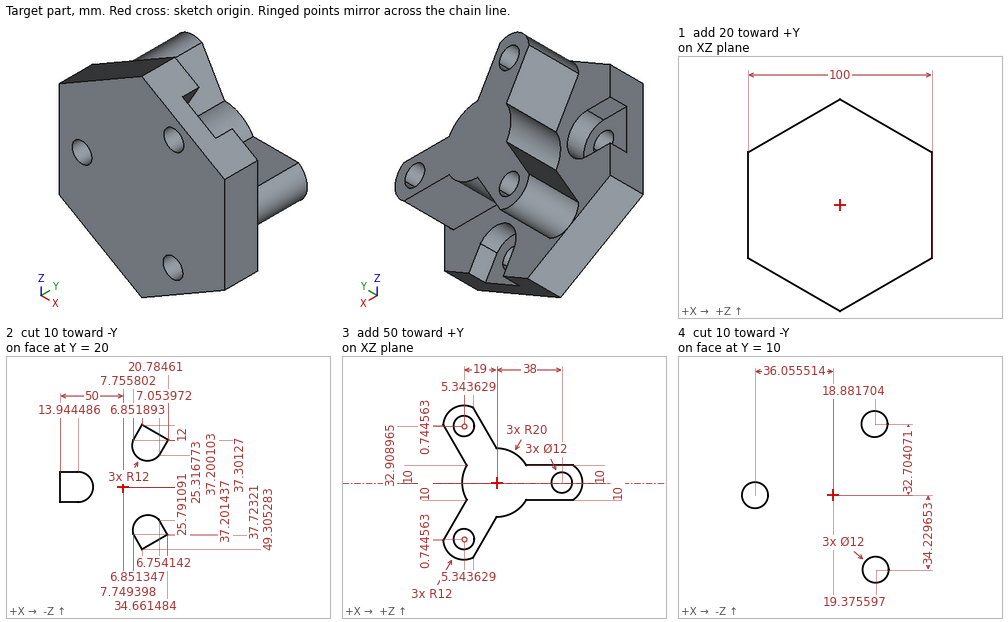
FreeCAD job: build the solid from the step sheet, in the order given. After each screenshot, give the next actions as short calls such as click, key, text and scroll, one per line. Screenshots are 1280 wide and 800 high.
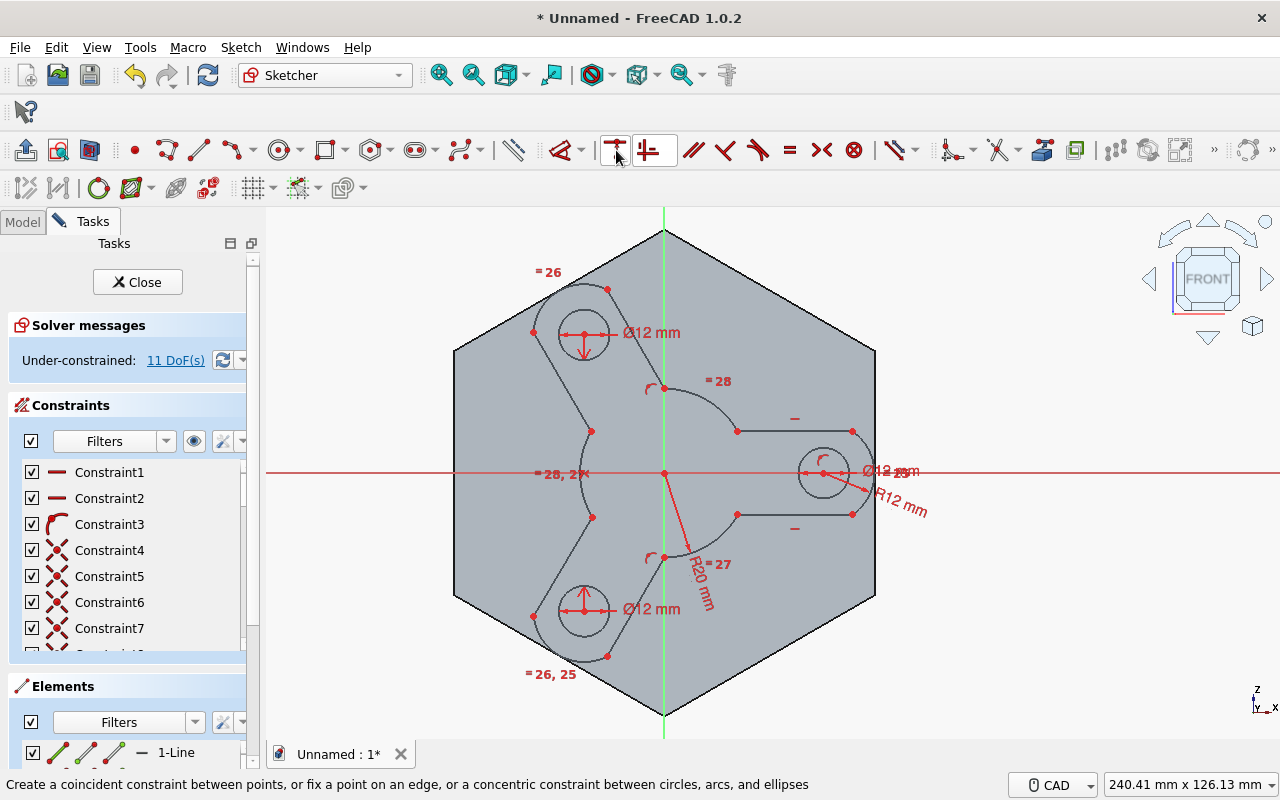
key(d)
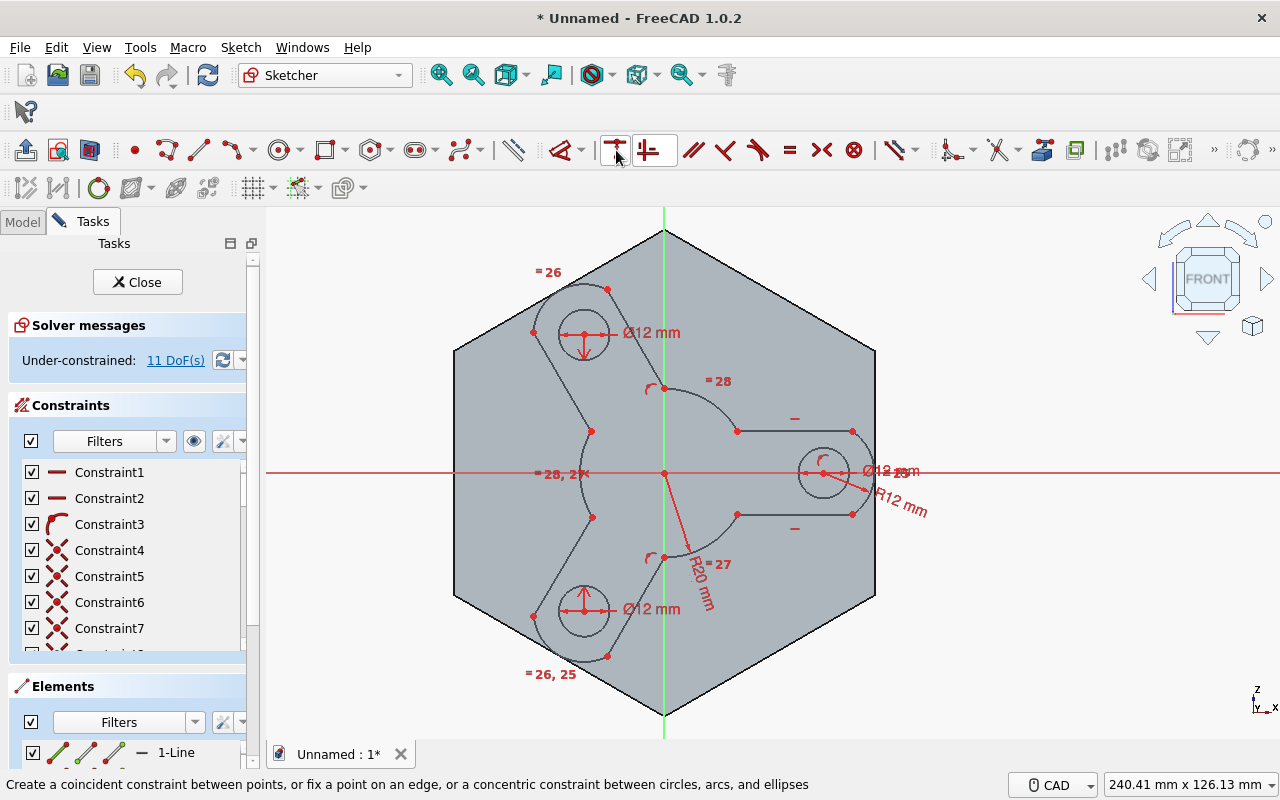
click(584, 335)
click(643, 301)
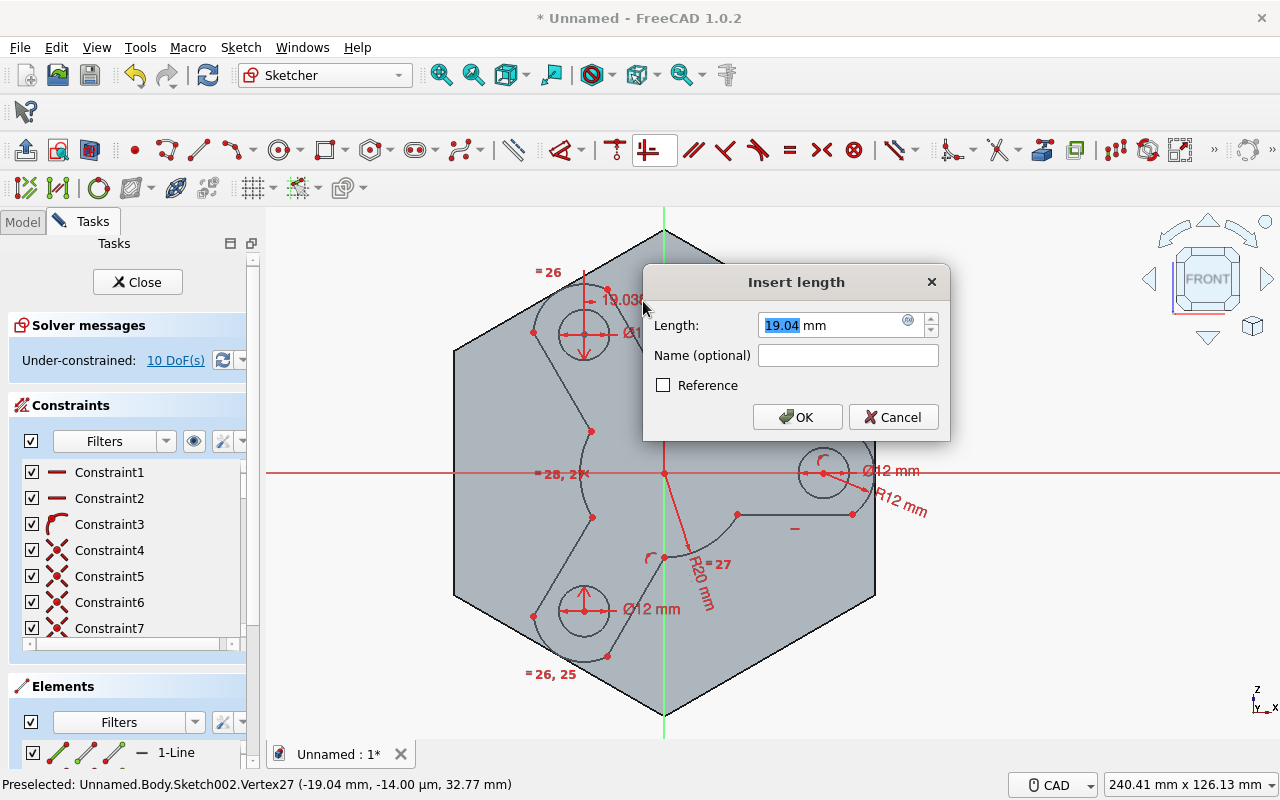
text(19)
key(Return)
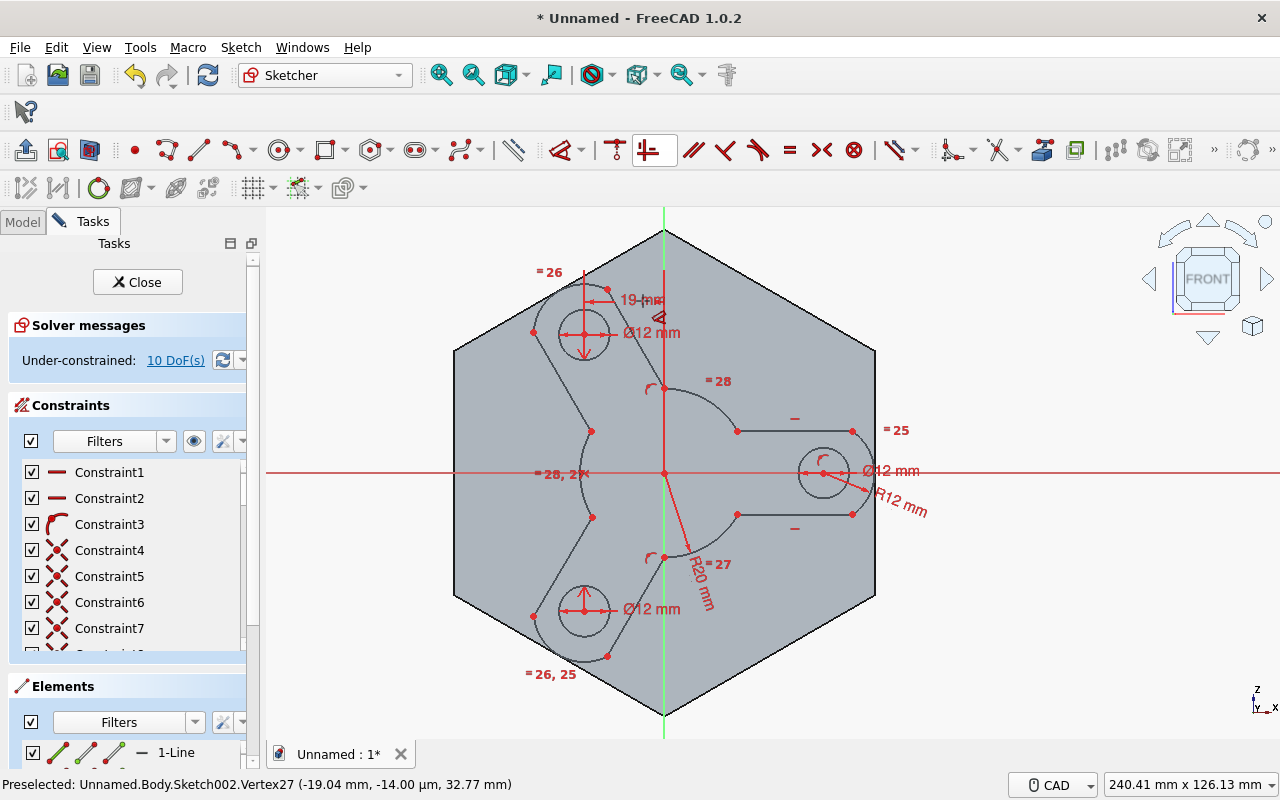
click(824, 473)
click(707, 507)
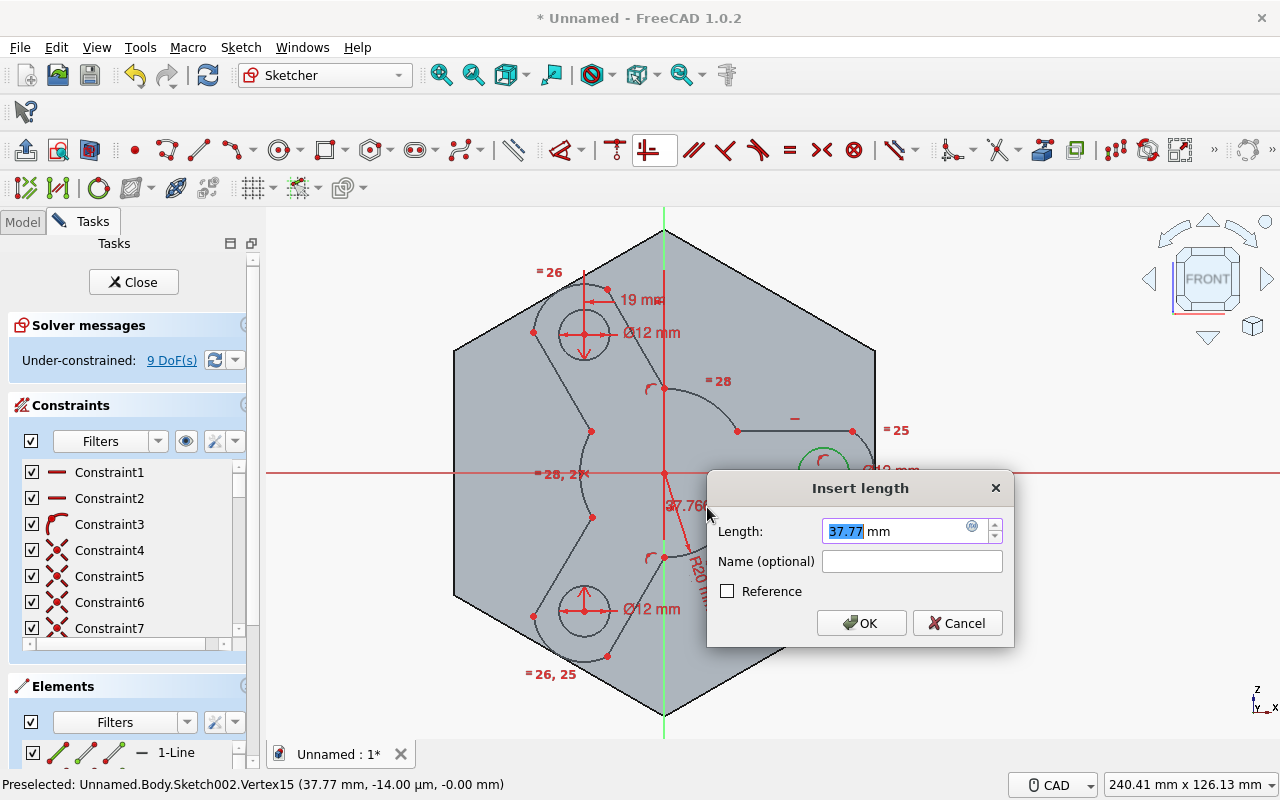
text(38)
key(Return)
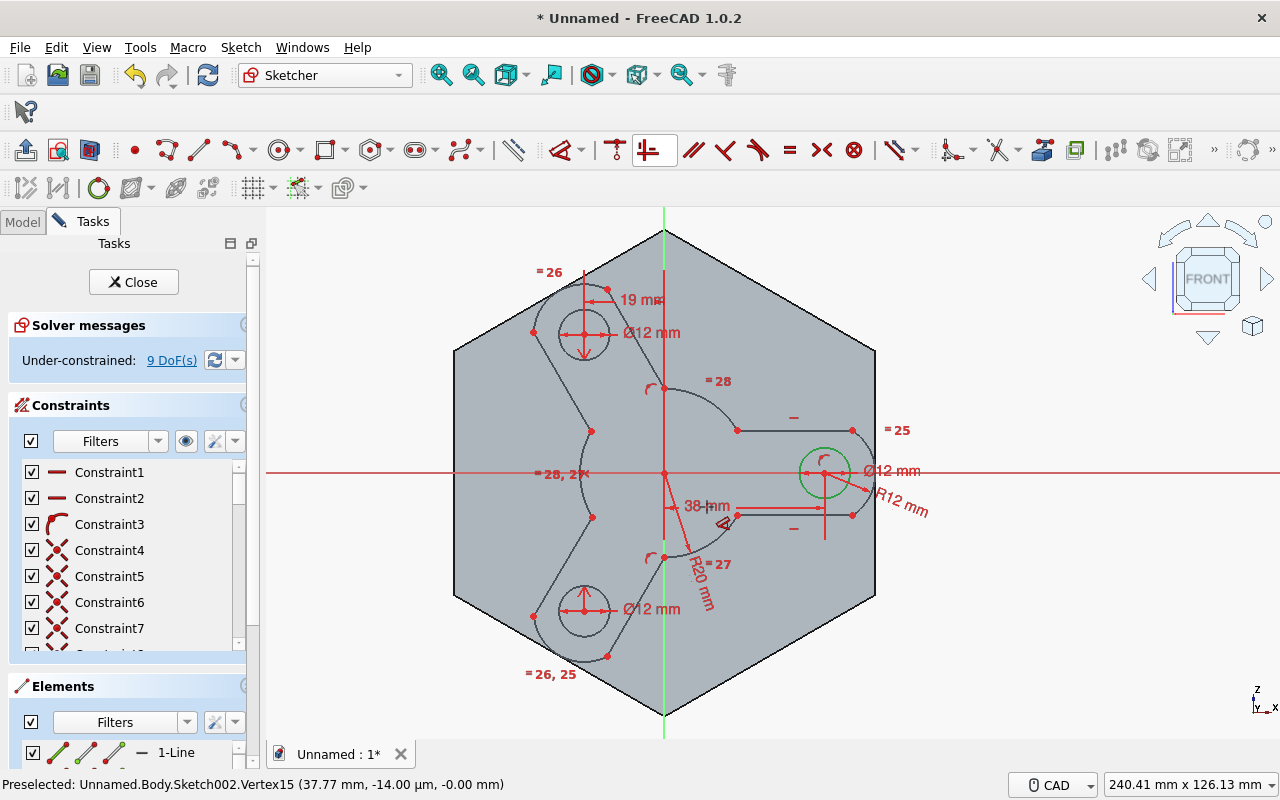
click(737, 431)
click(630, 452)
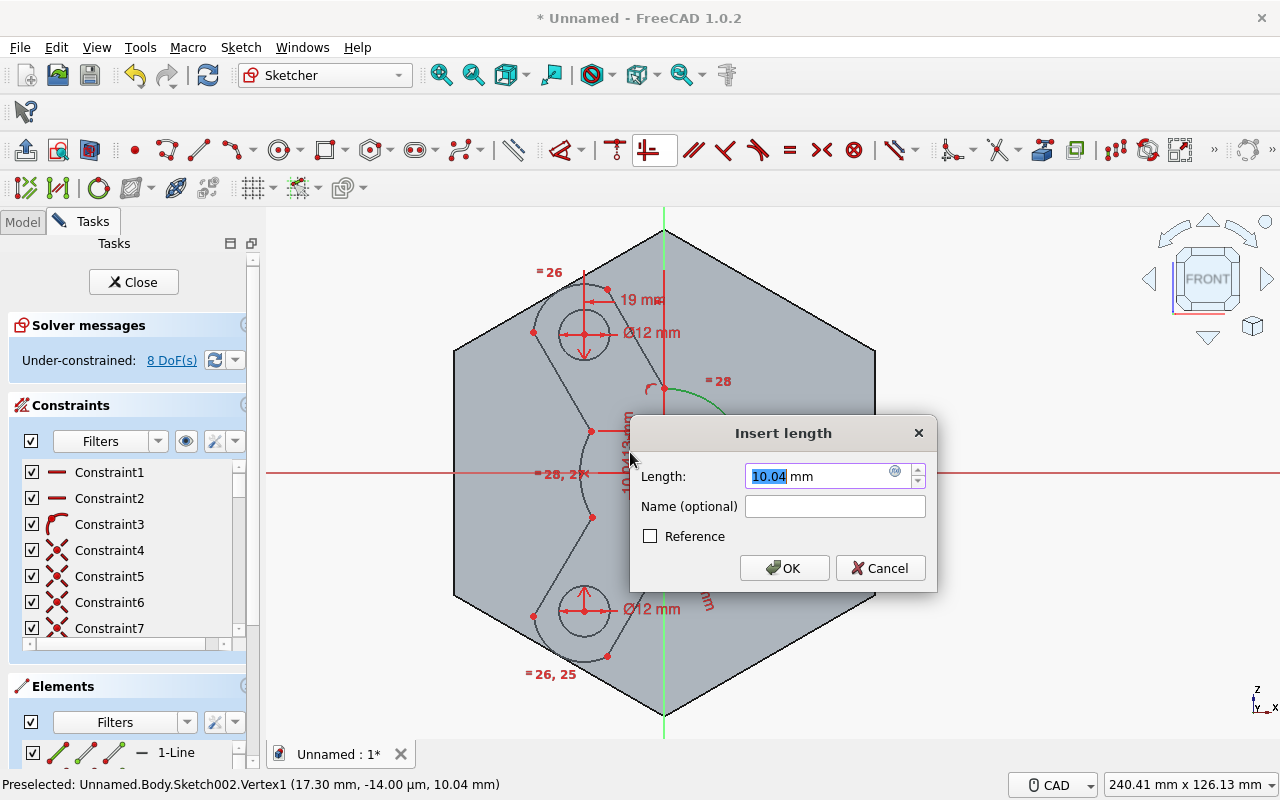
text(10)
key(Return)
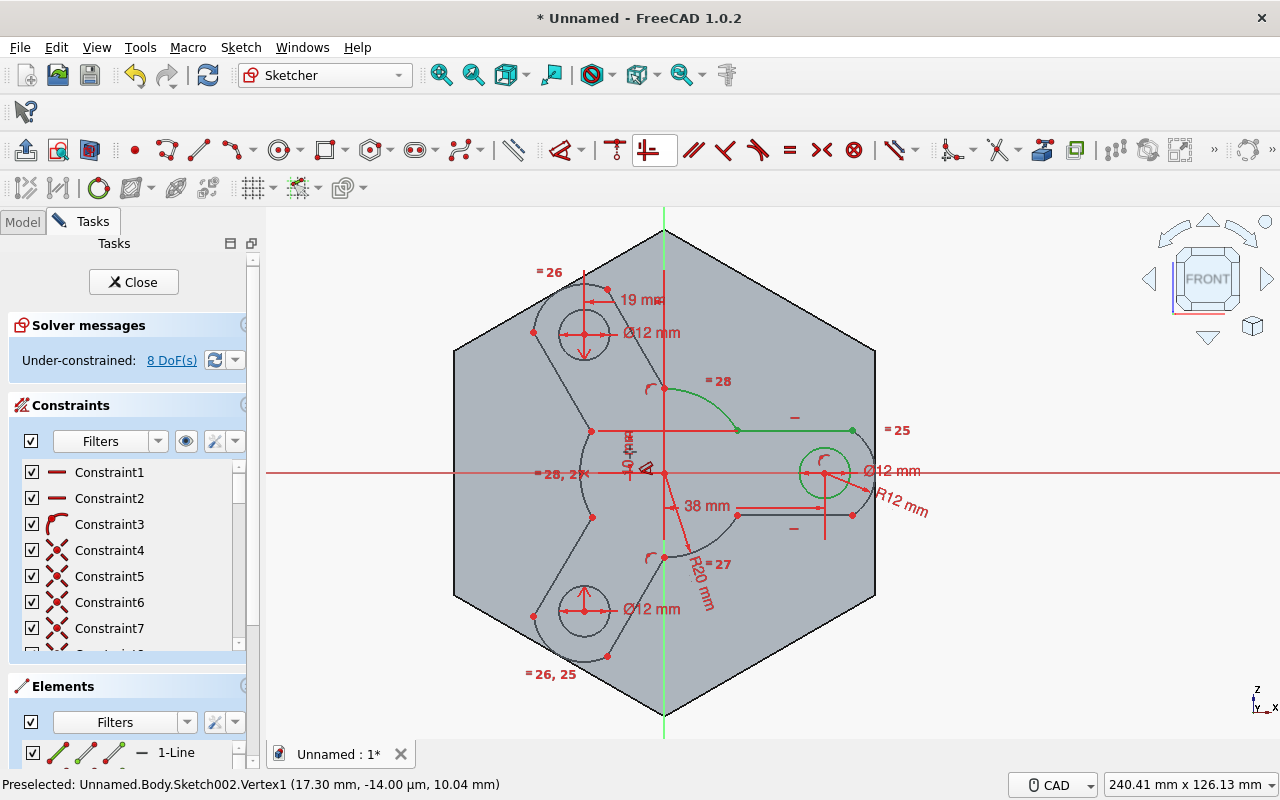
click(852, 515)
click(630, 494)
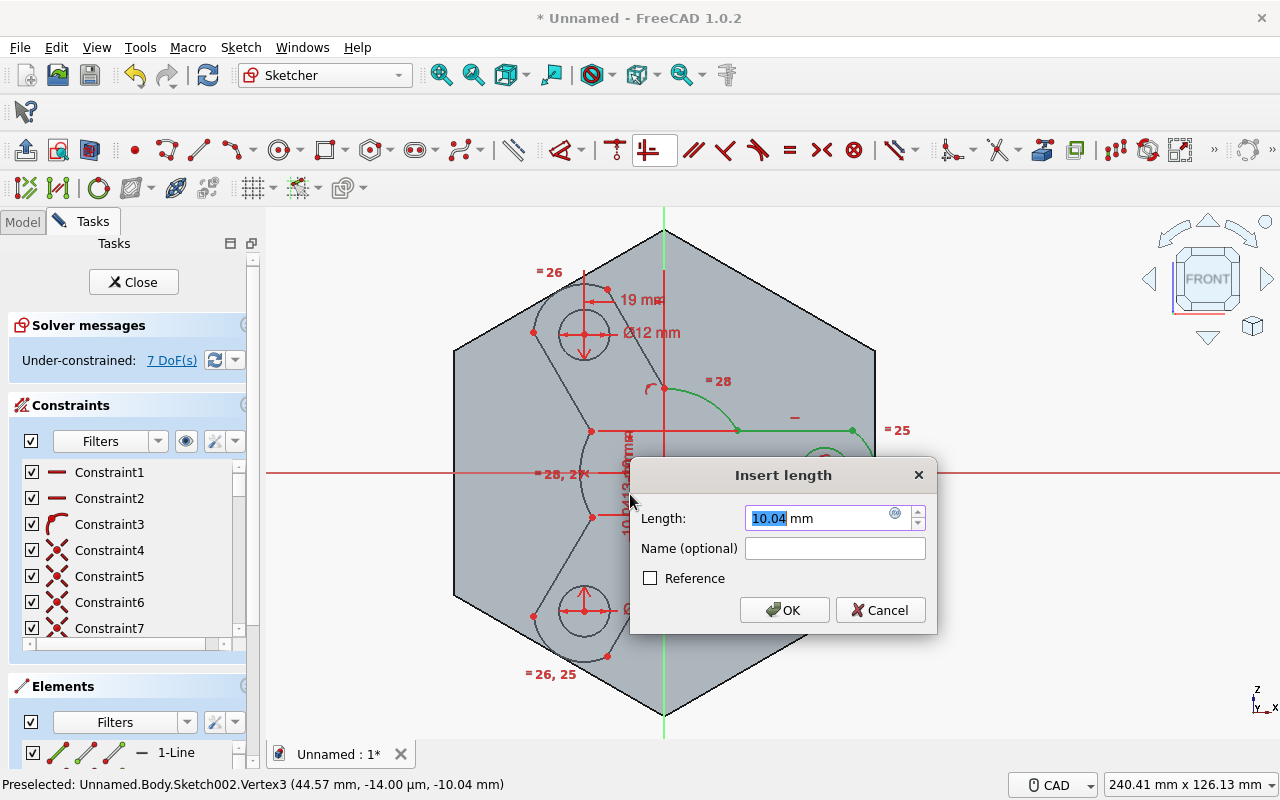
text(10)
key(Return)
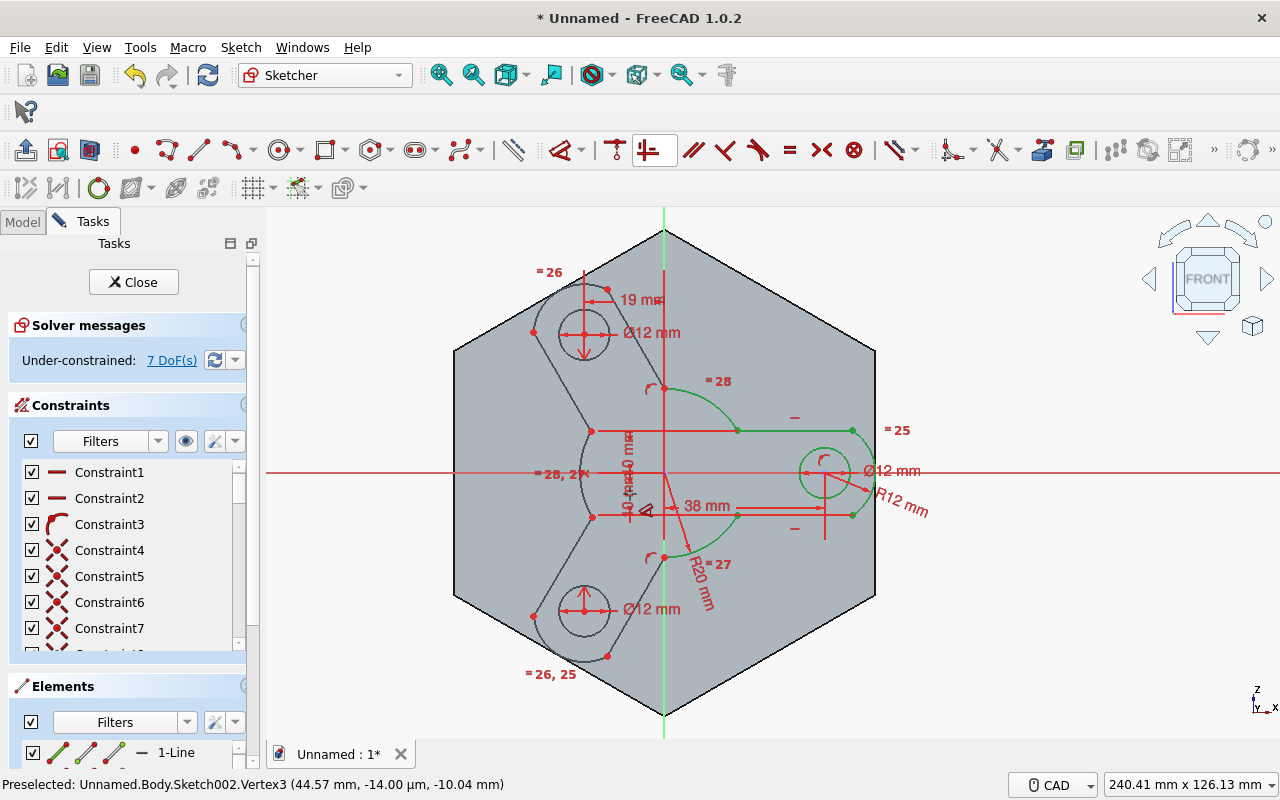
click(592, 517)
click(558, 495)